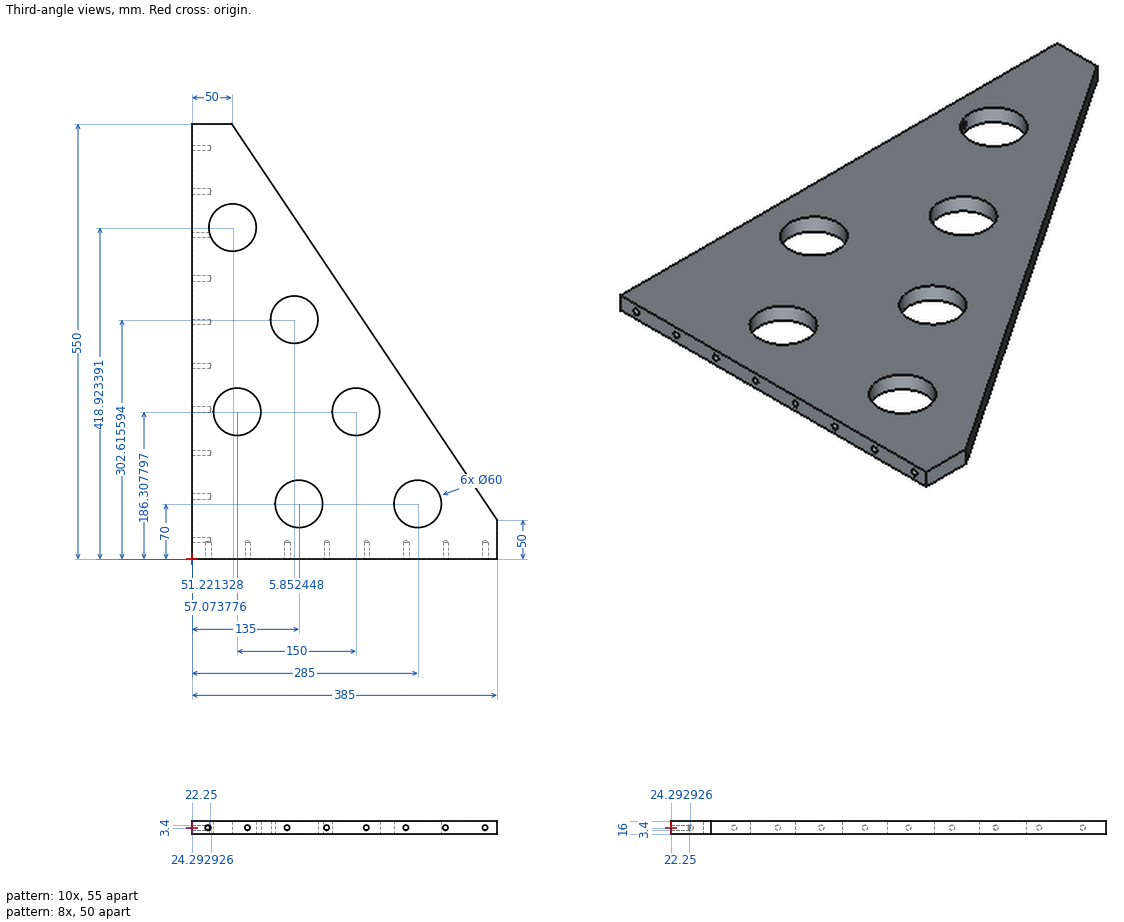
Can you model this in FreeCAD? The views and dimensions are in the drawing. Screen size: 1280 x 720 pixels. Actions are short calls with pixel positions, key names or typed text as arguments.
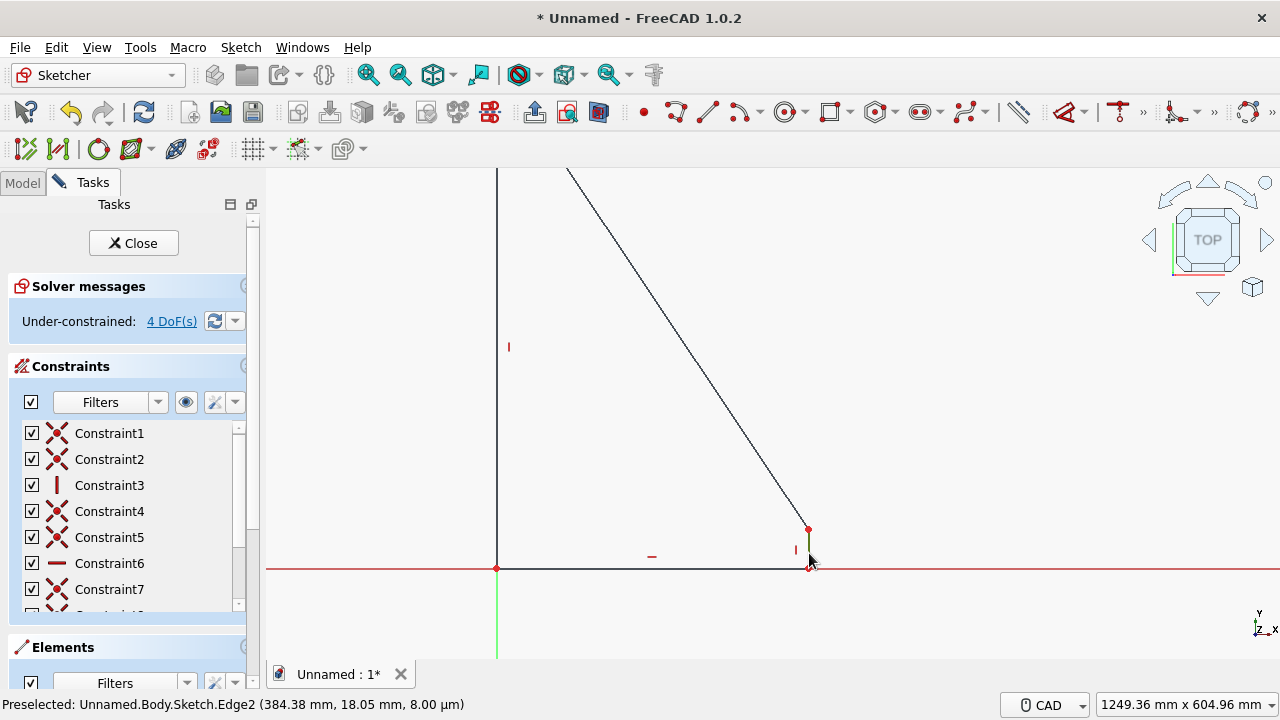
key(i)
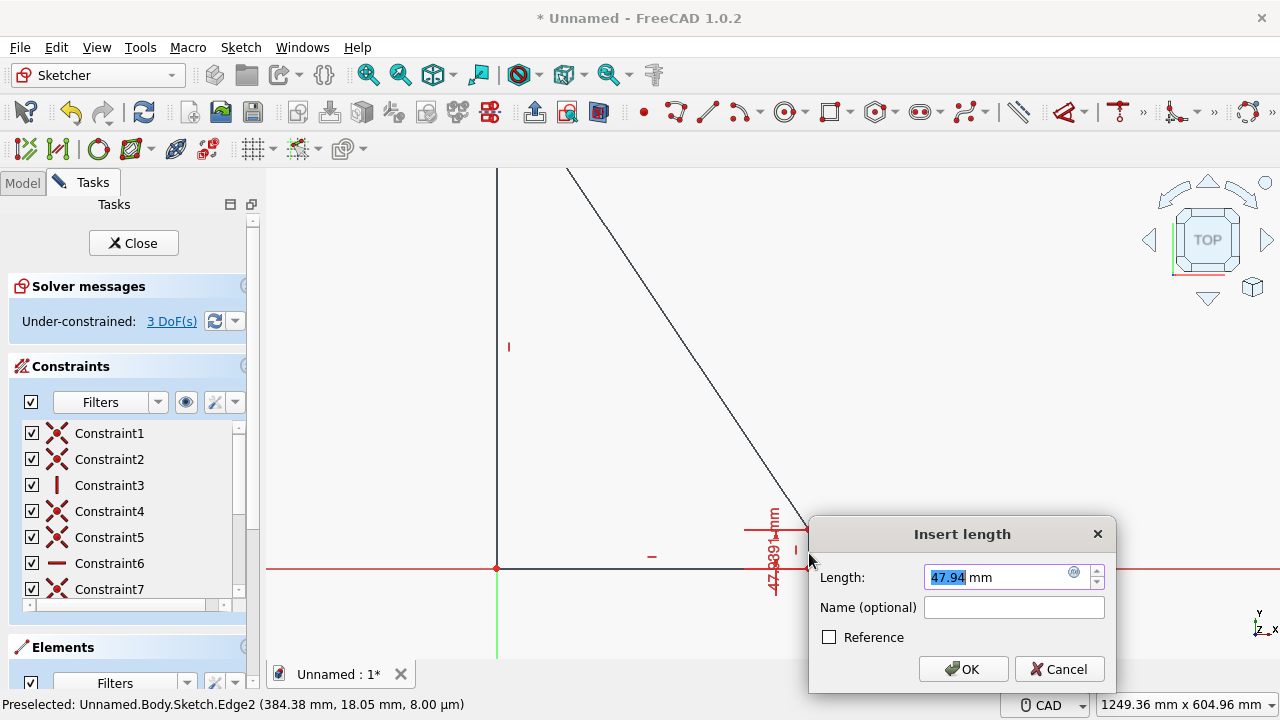
text(50)
key(Return)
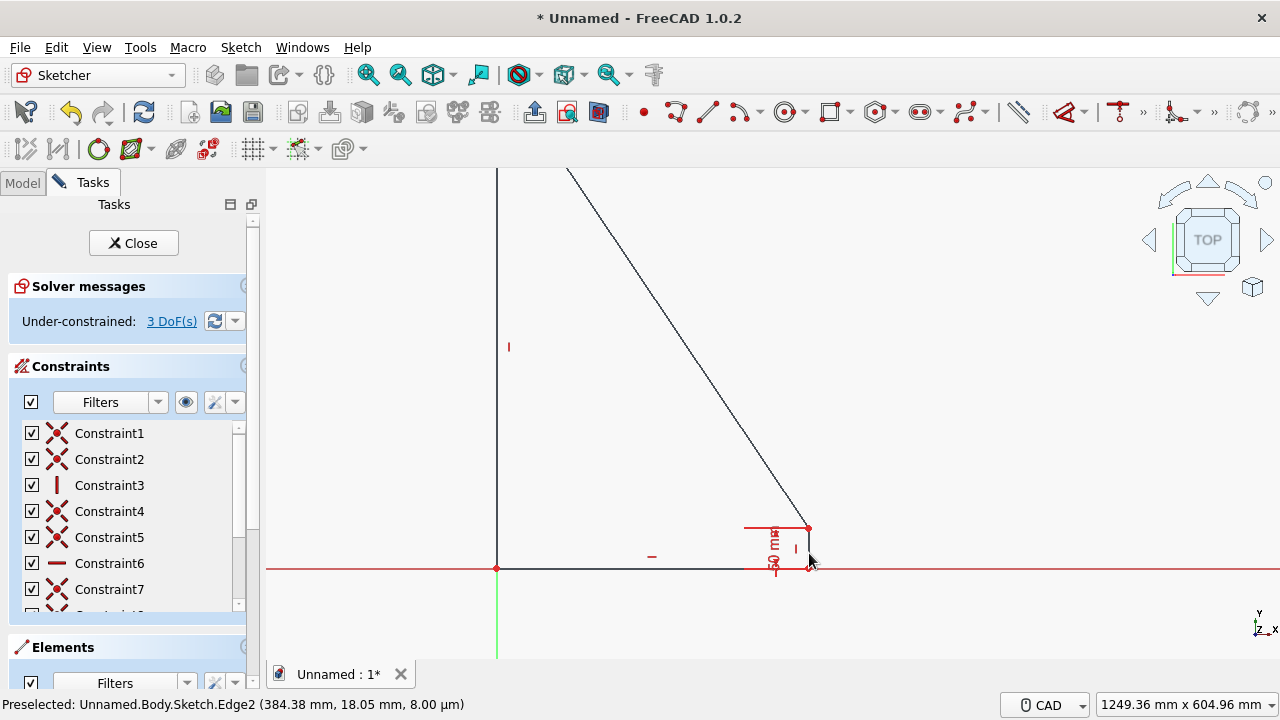
scroll(809, 552, down, 2)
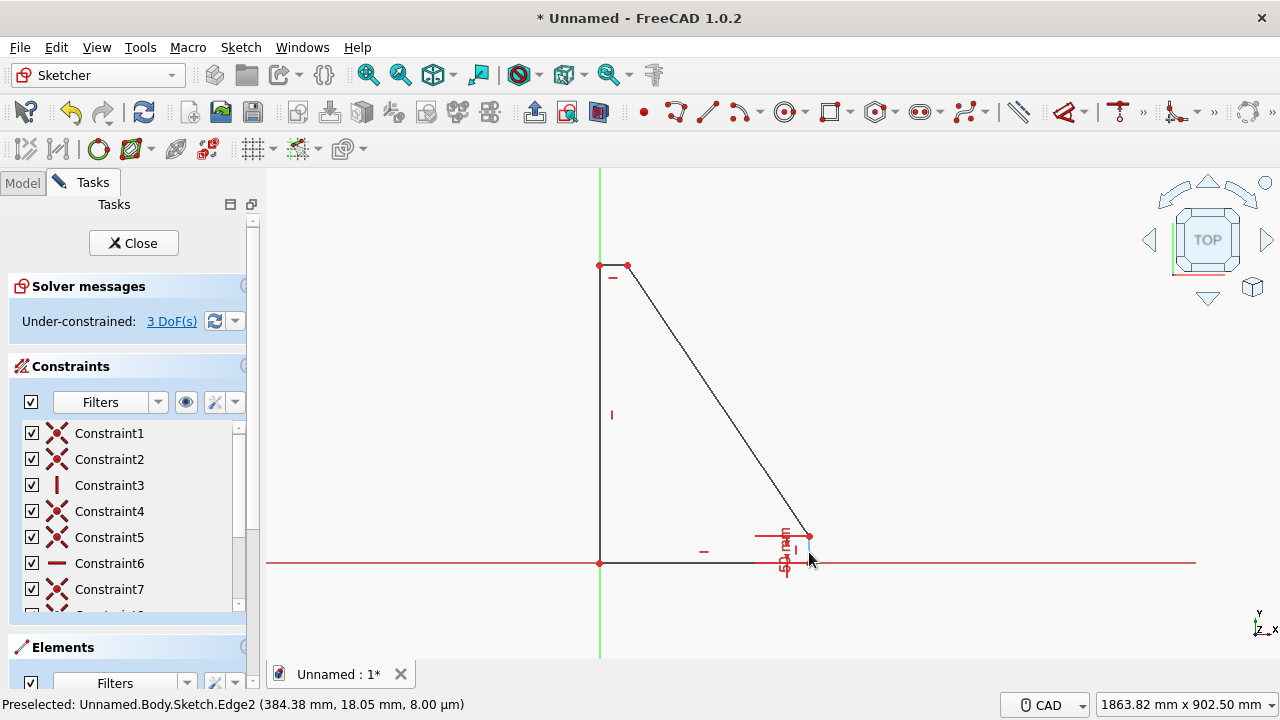
scroll(619, 265, up, 3)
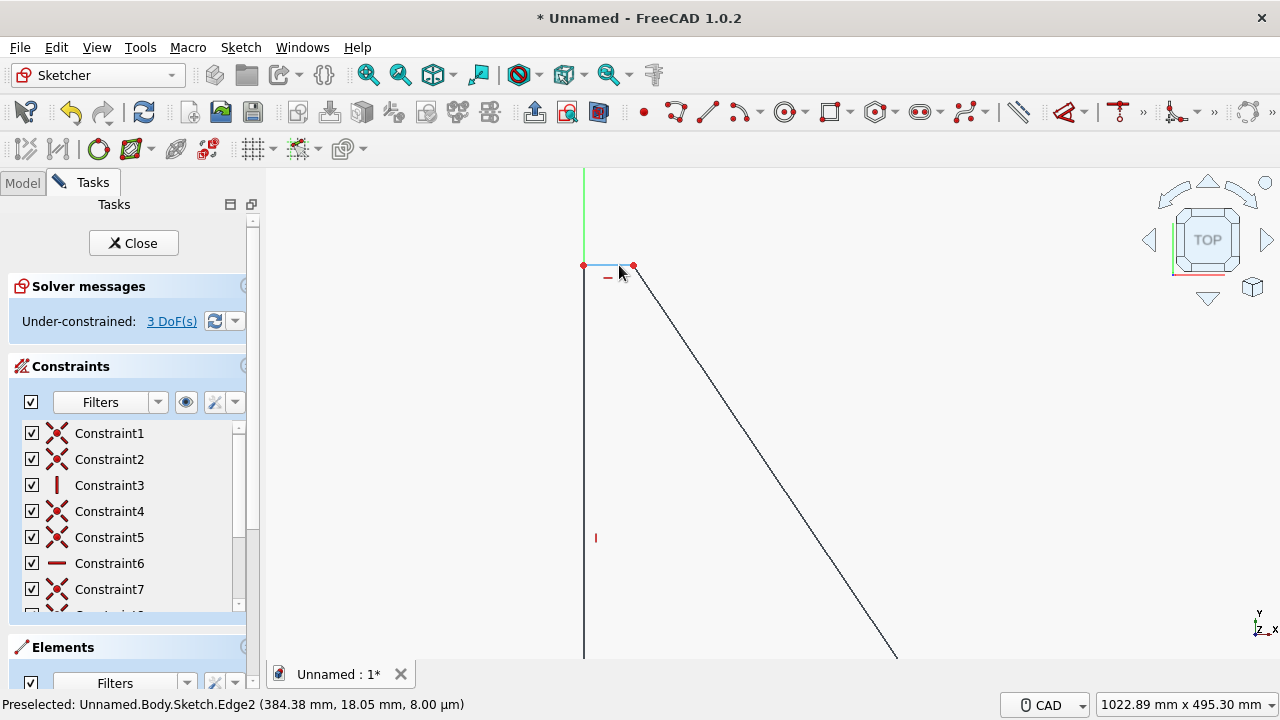
click(618, 265)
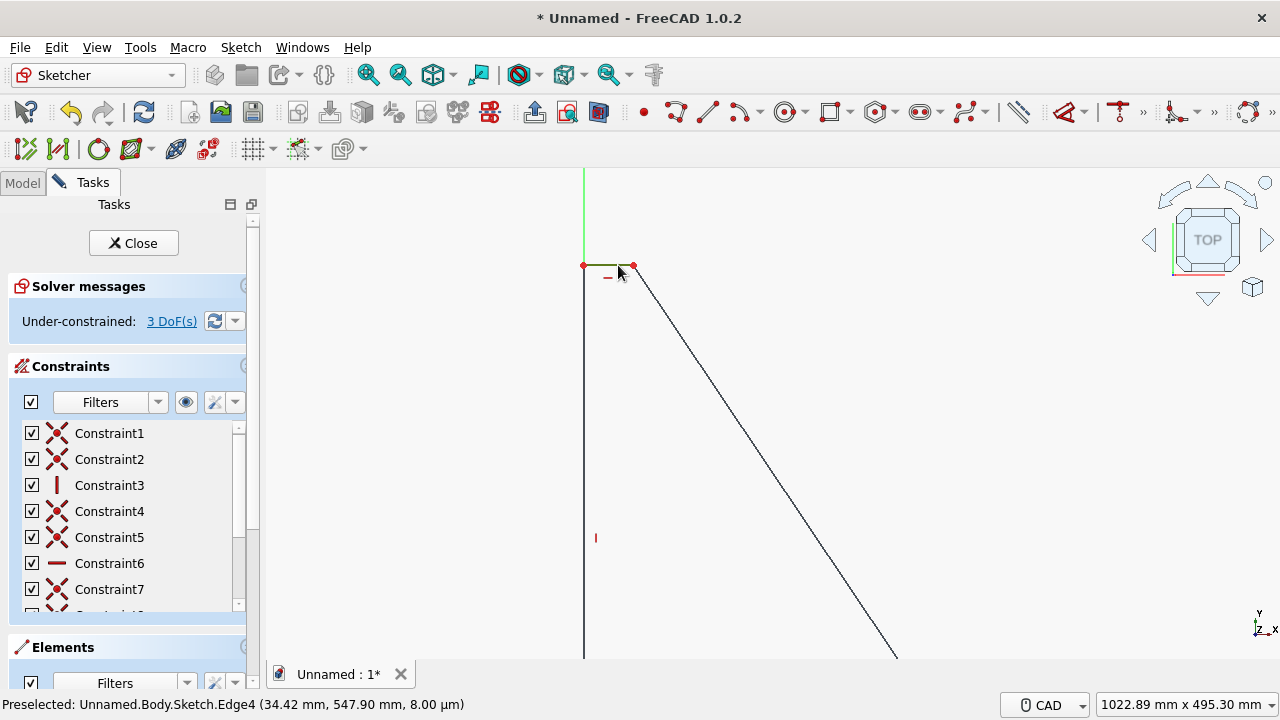
click(1086, 112)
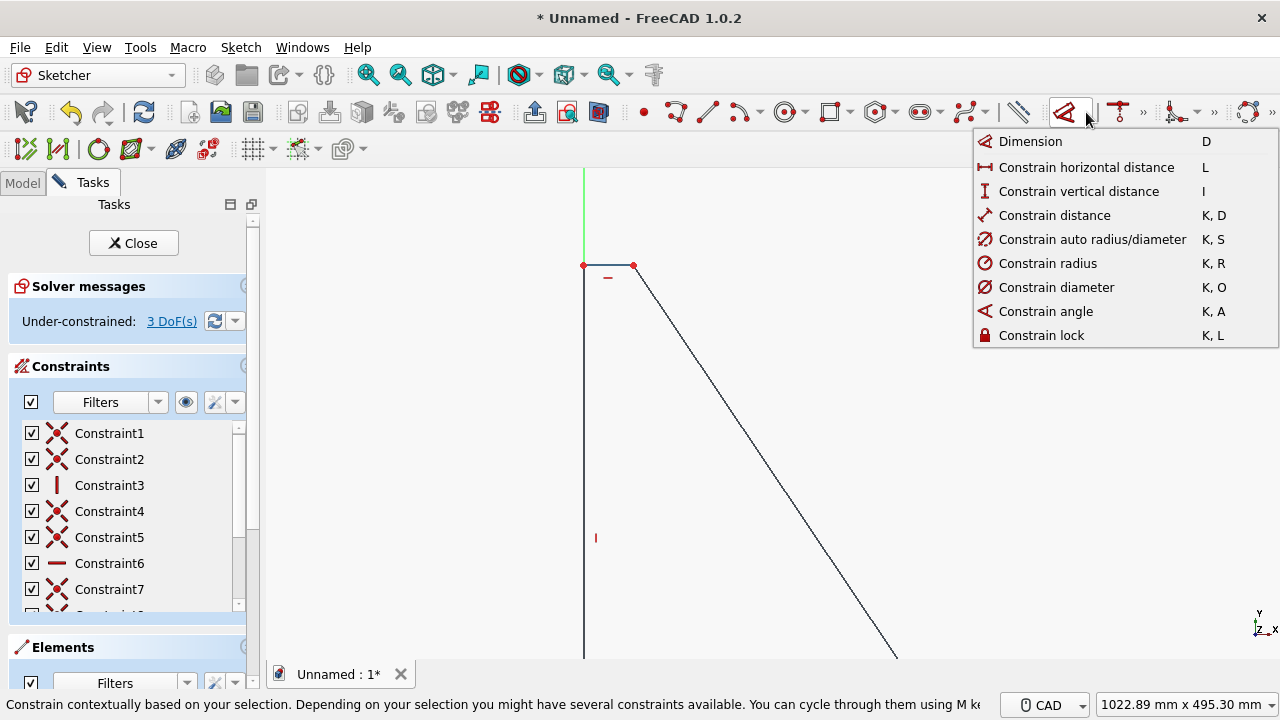
click(1126, 167)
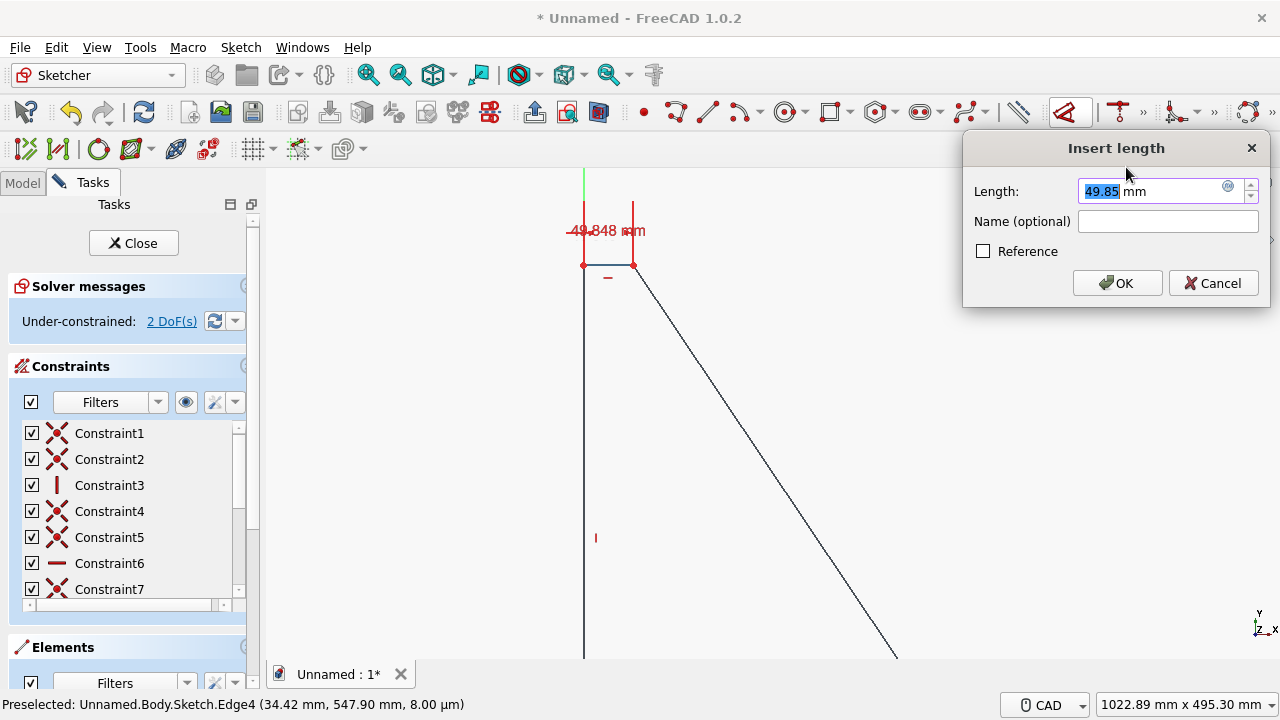
text(50)
key(Return)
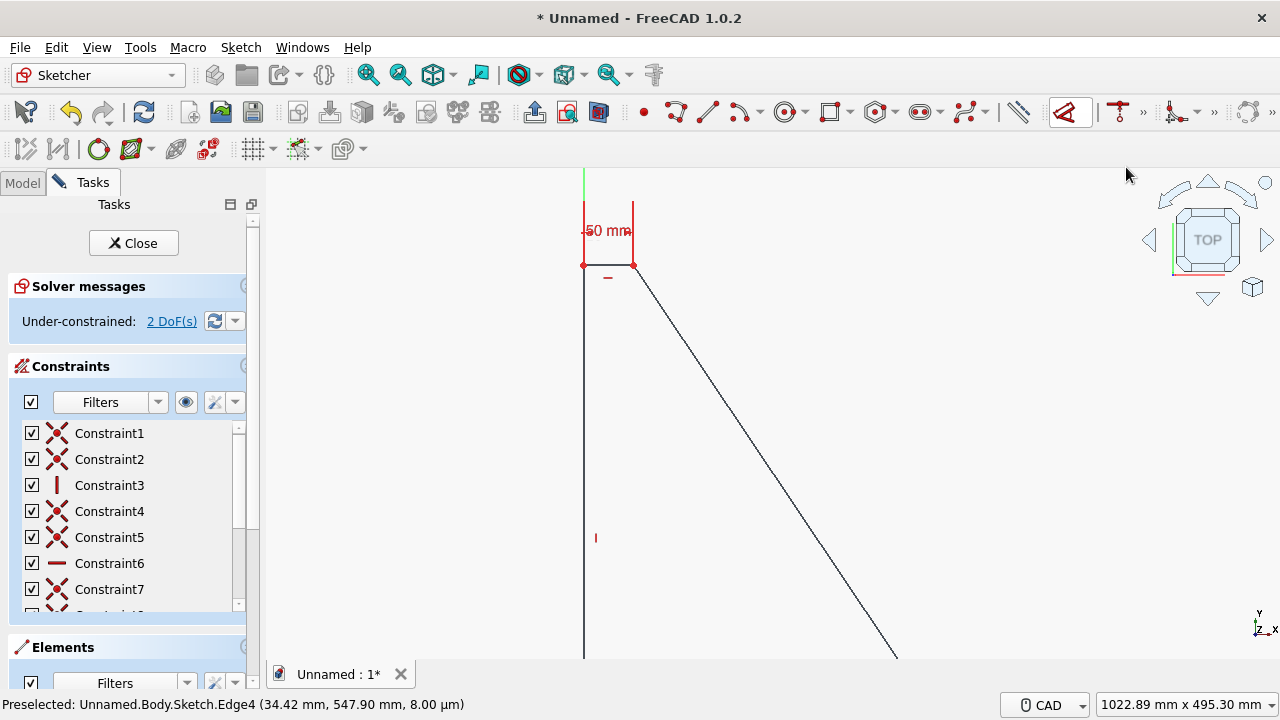
scroll(619, 265, down, 3)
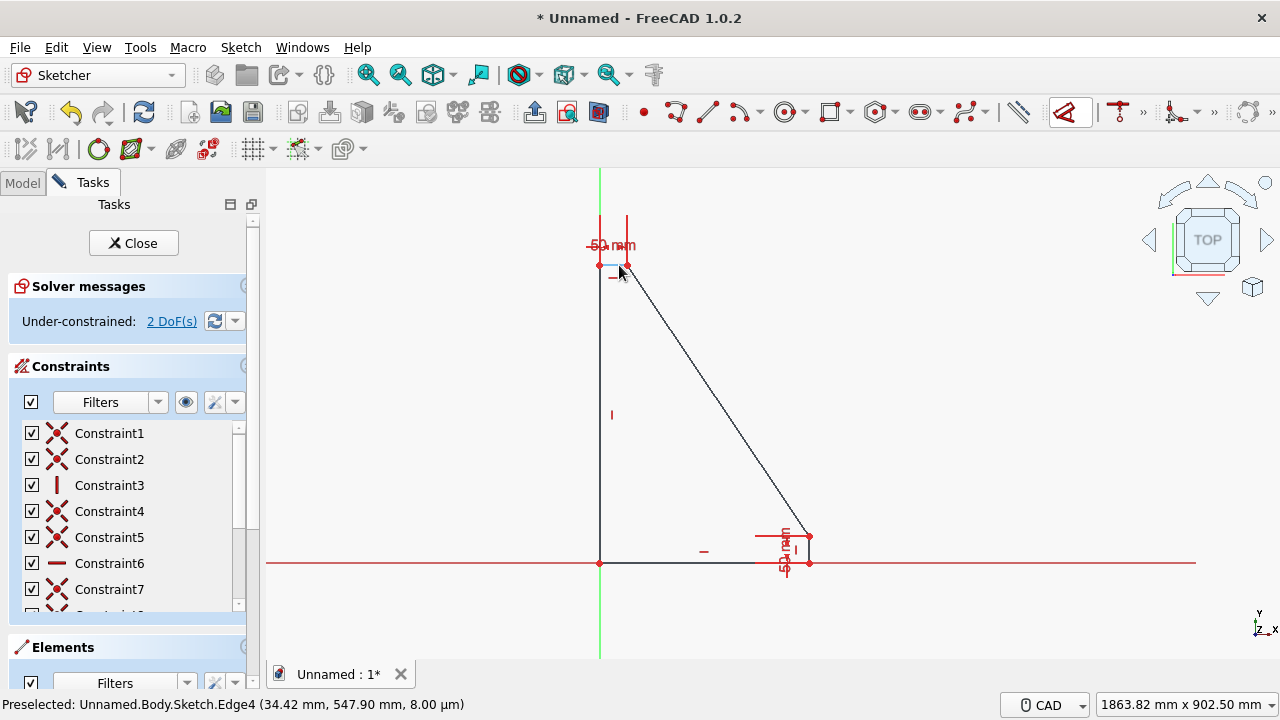
click(663, 563)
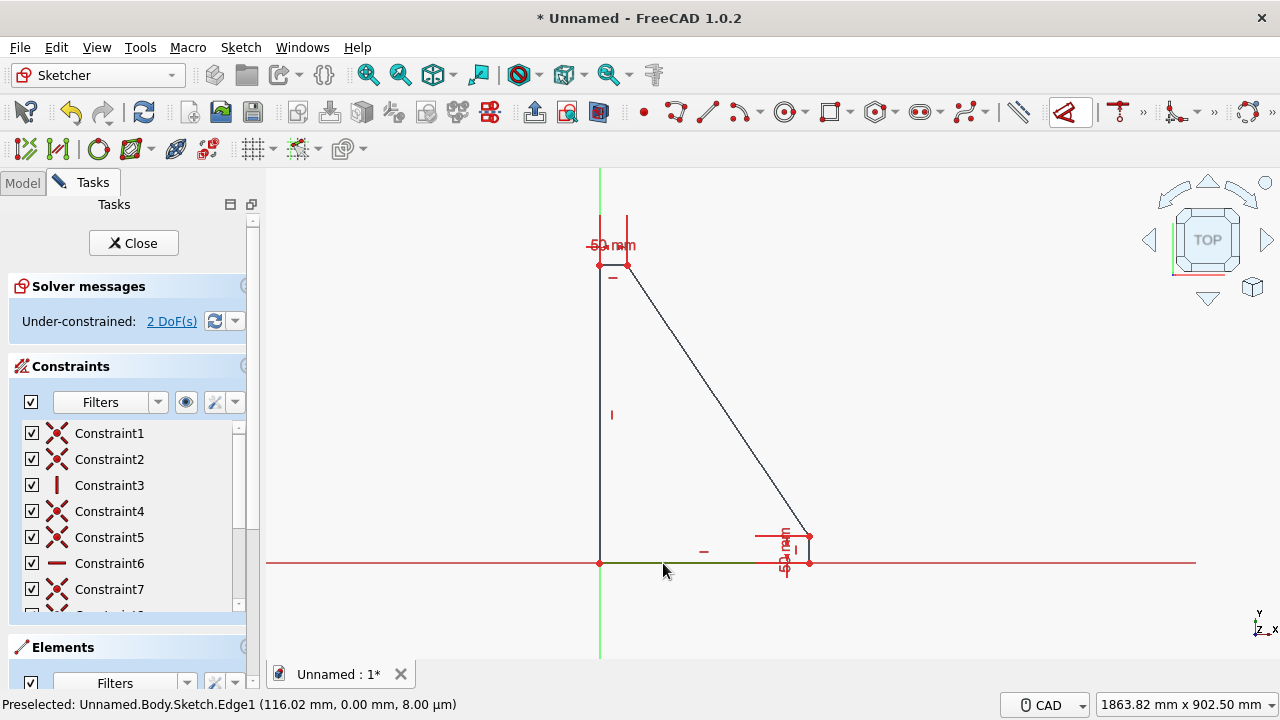
key(l)